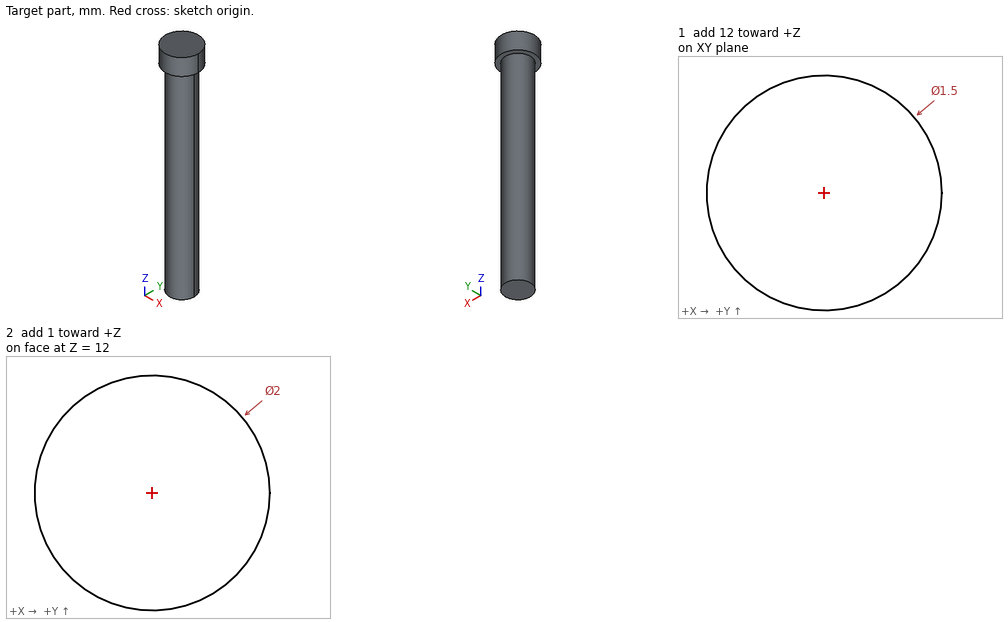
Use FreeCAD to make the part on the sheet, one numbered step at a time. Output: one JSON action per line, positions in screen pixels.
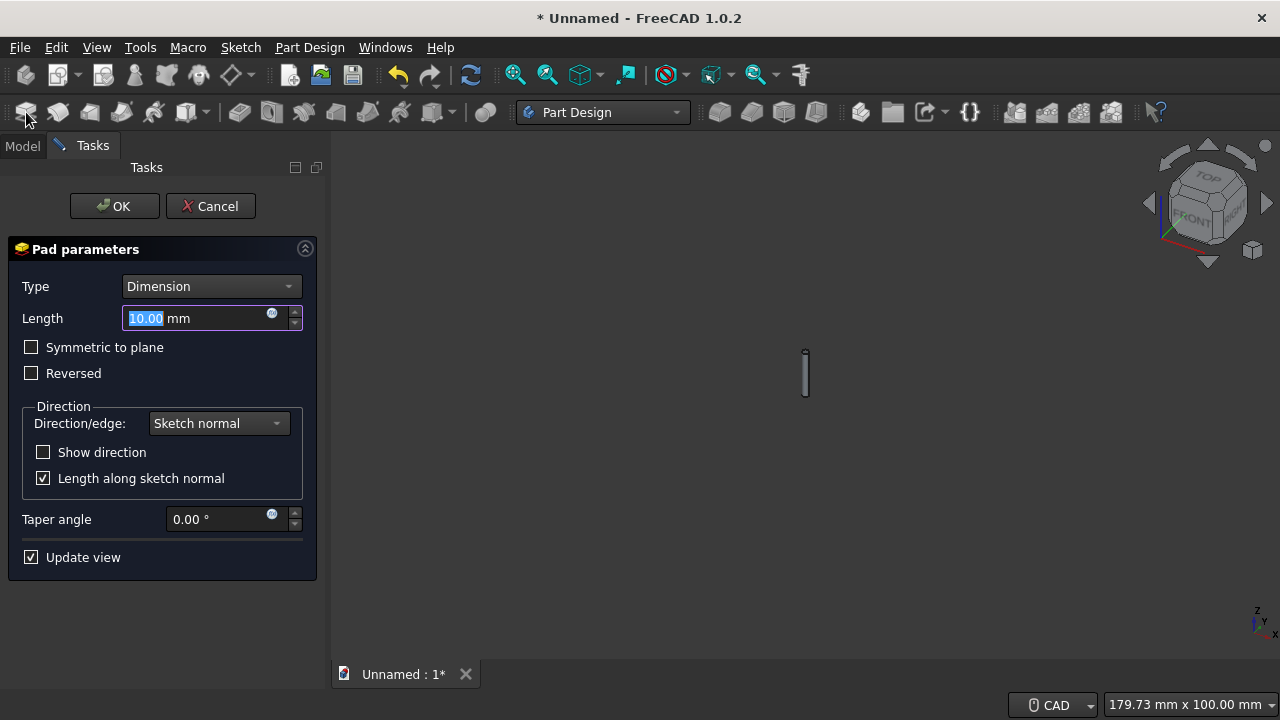
{"action": "type", "text": "12"}
{"action": "key", "text": "Tab"}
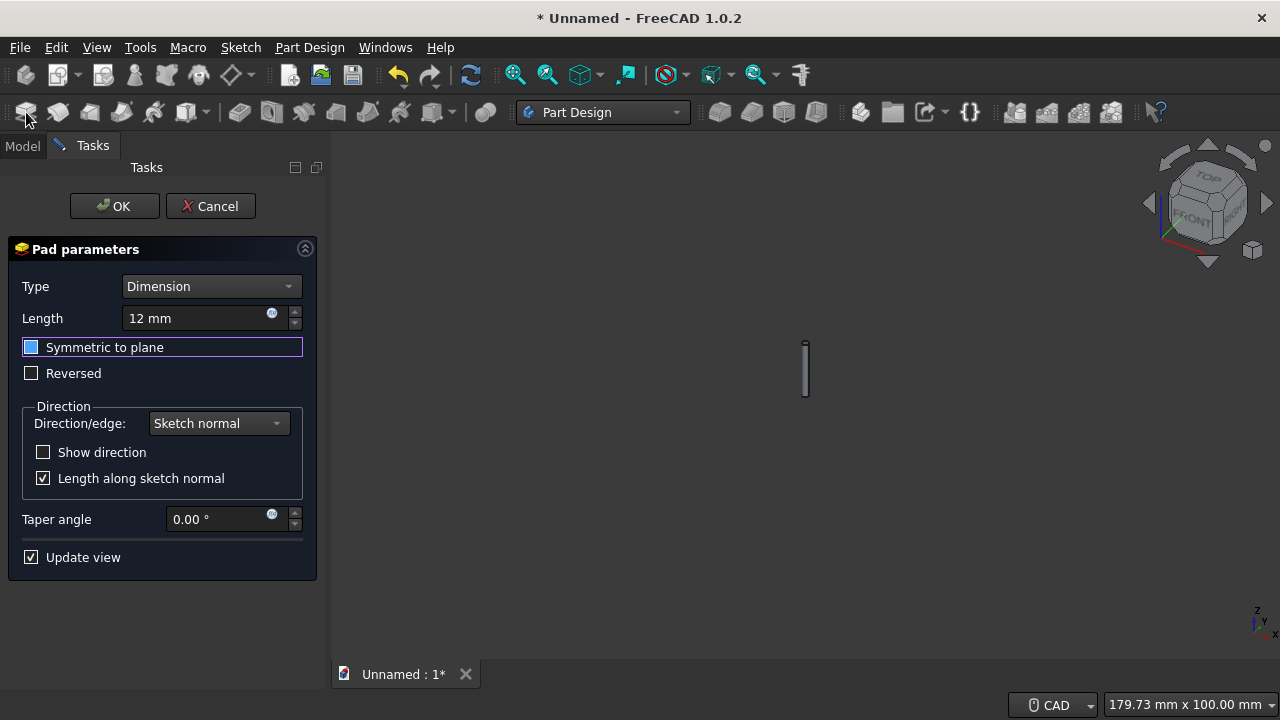
{"action": "left_click", "coordinate": [115, 206]}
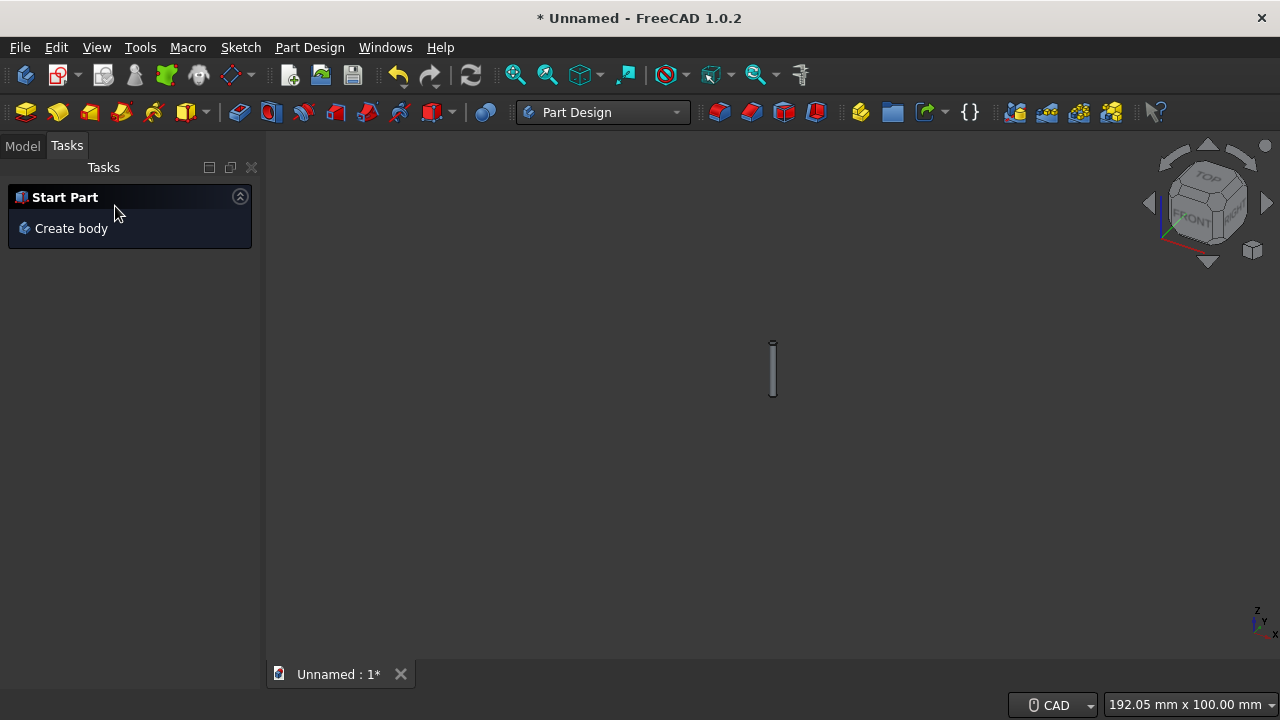
{"action": "left_click", "coordinate": [516, 76]}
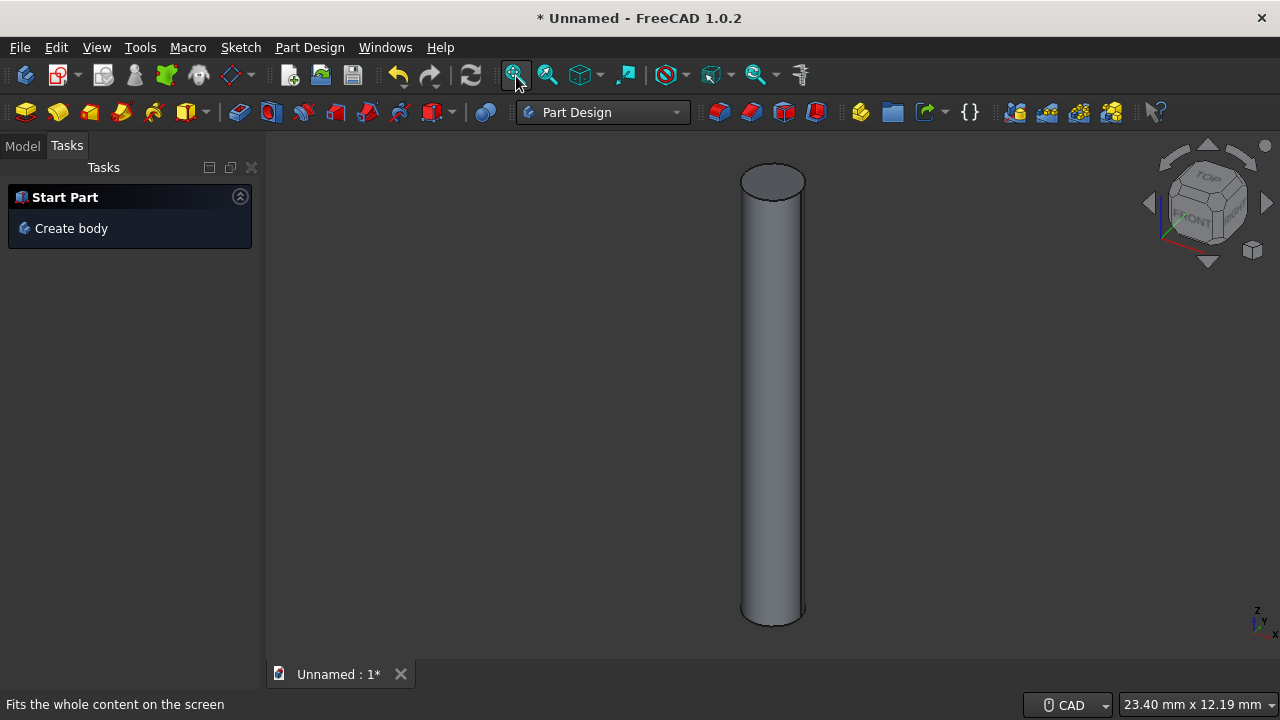
{"action": "left_click", "coordinate": [773, 181]}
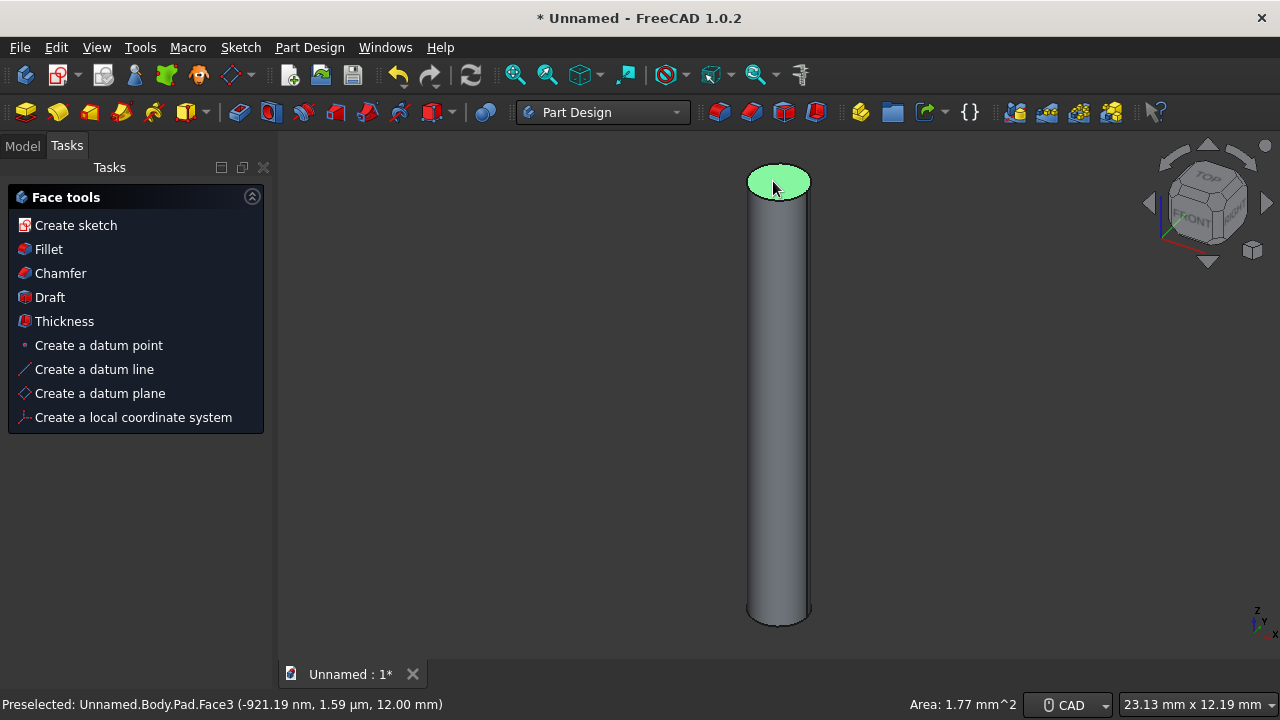
{"action": "left_click", "coordinate": [58, 76]}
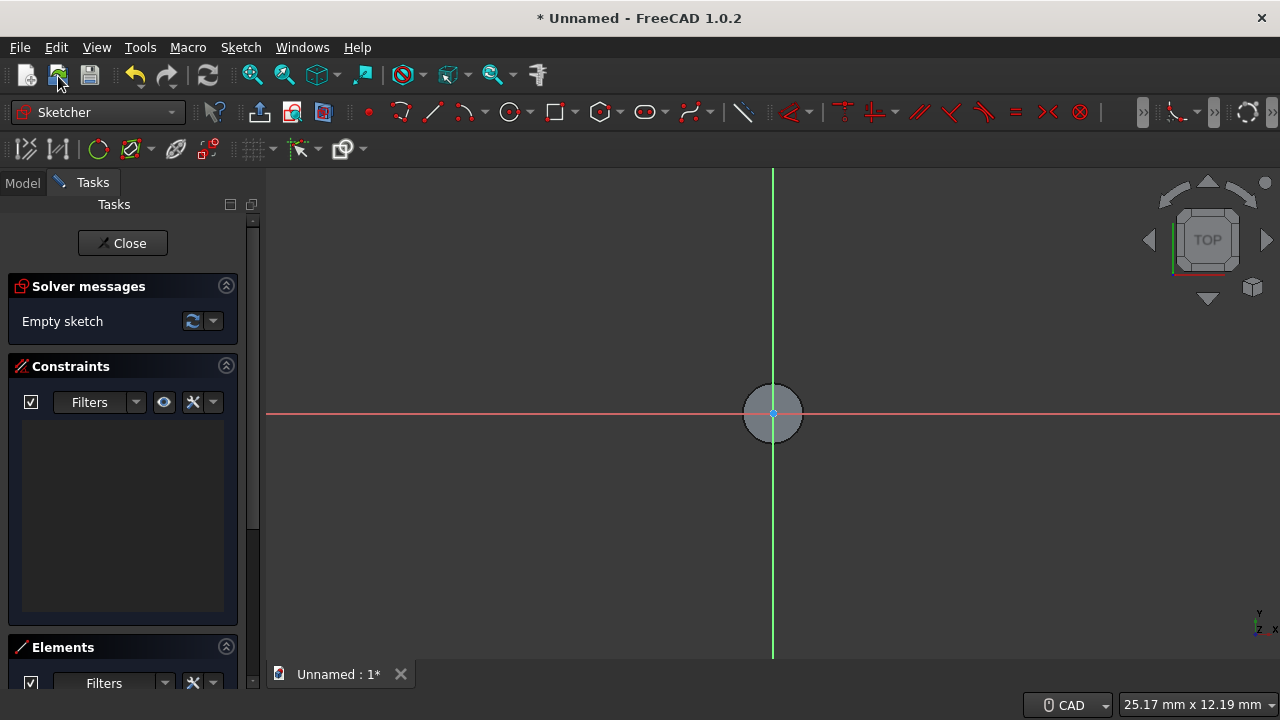
{"action": "scroll", "coordinate": [795, 414], "scroll_direction": "up", "scroll_amount": 7}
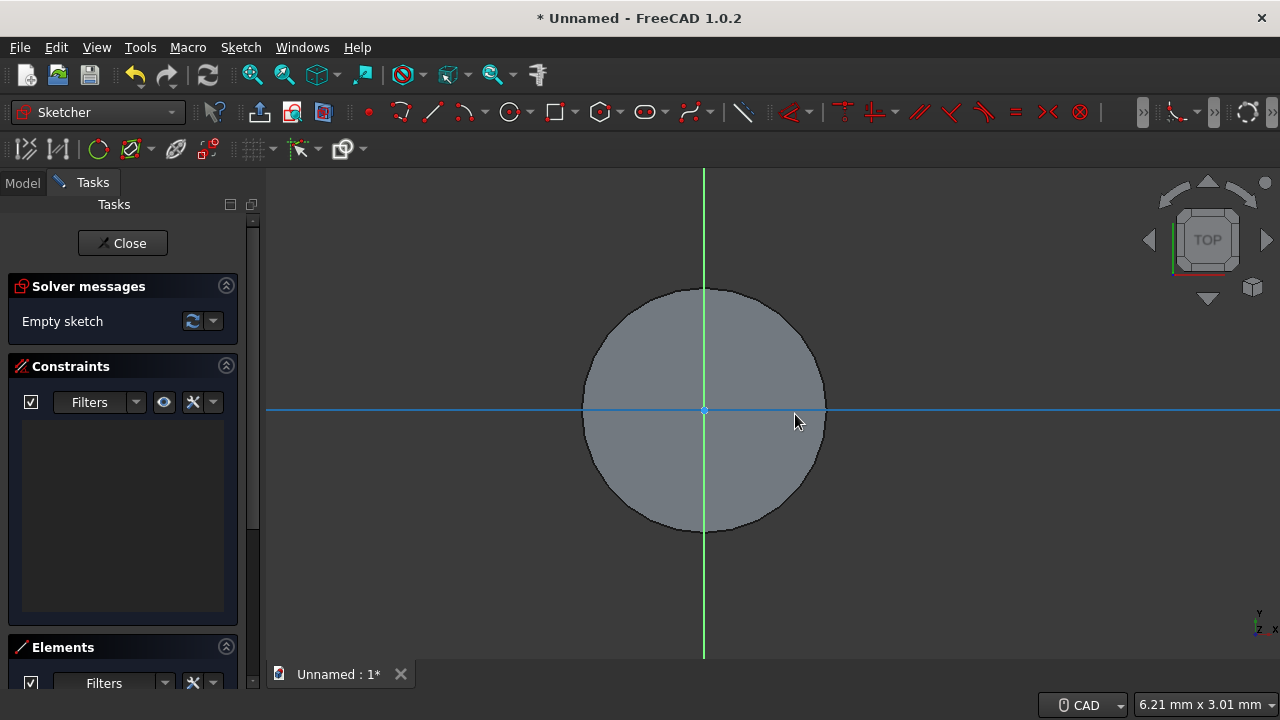
{"action": "left_click", "coordinate": [510, 112]}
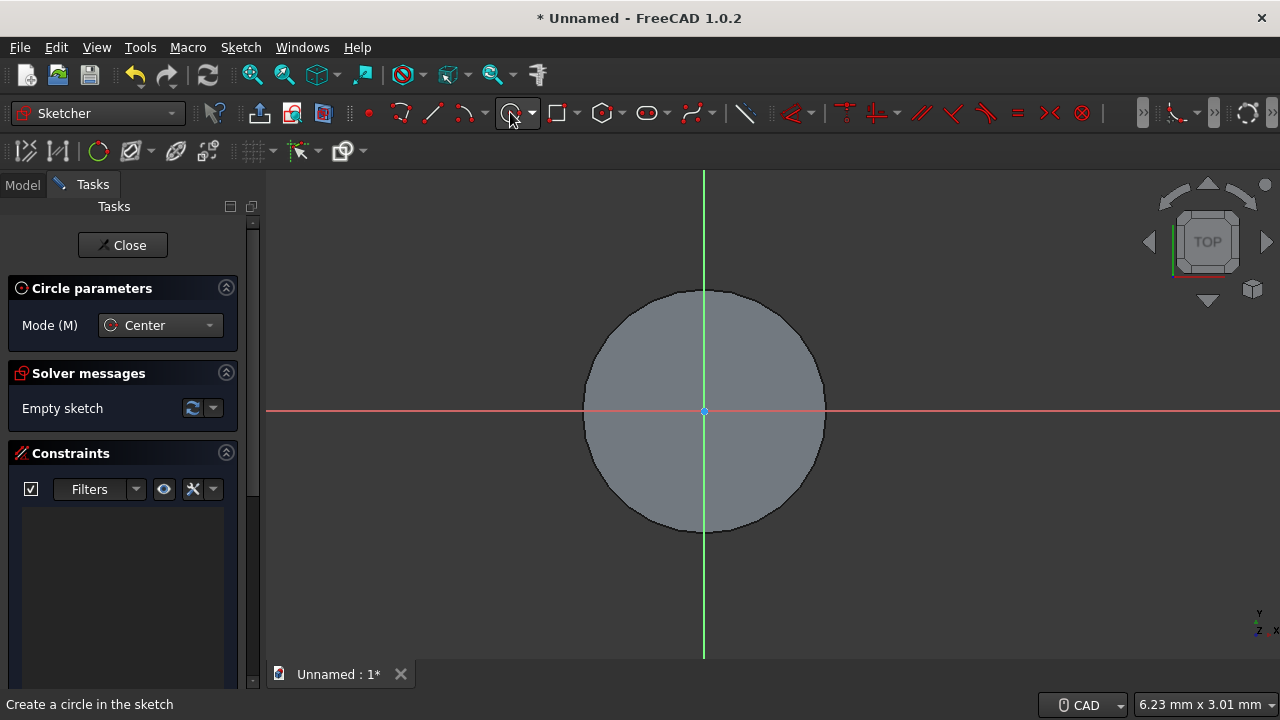
{"action": "left_click", "coordinate": [704, 411]}
{"action": "mouse_move", "coordinate": [820, 296]}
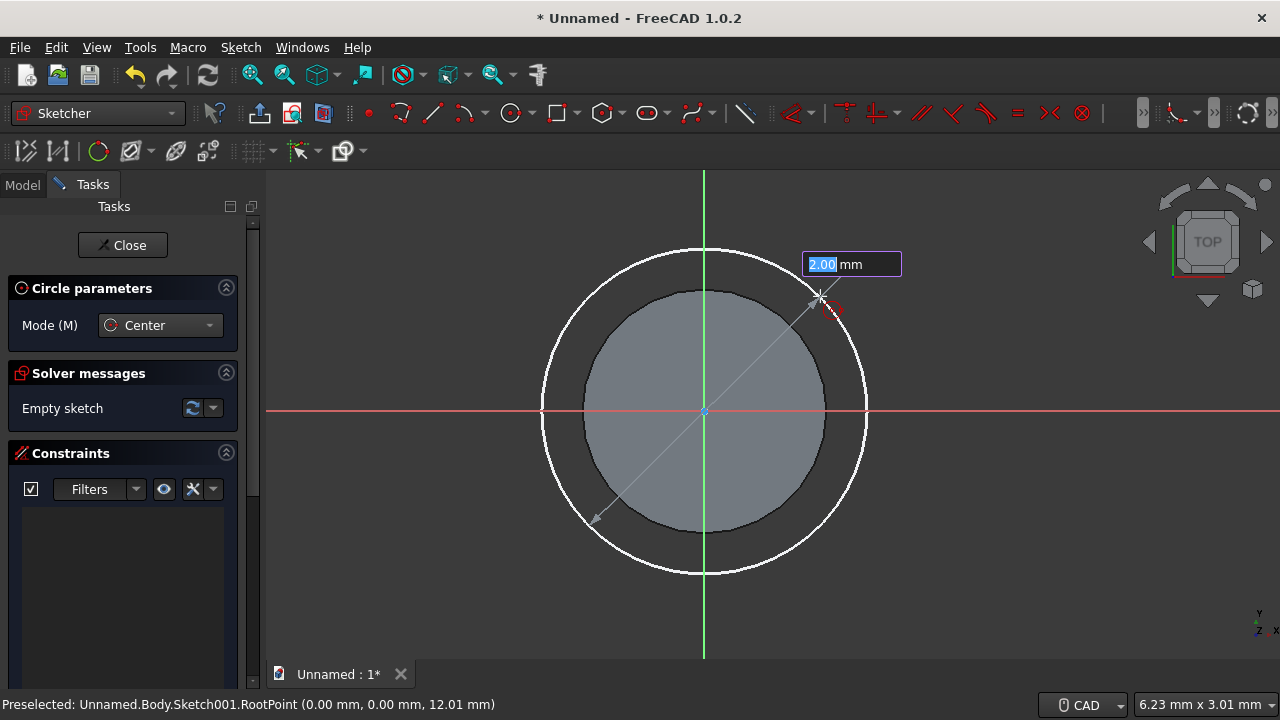
{"action": "type", "text": "2"}
{"action": "key", "text": "Return"}
{"action": "key", "text": "Escape"}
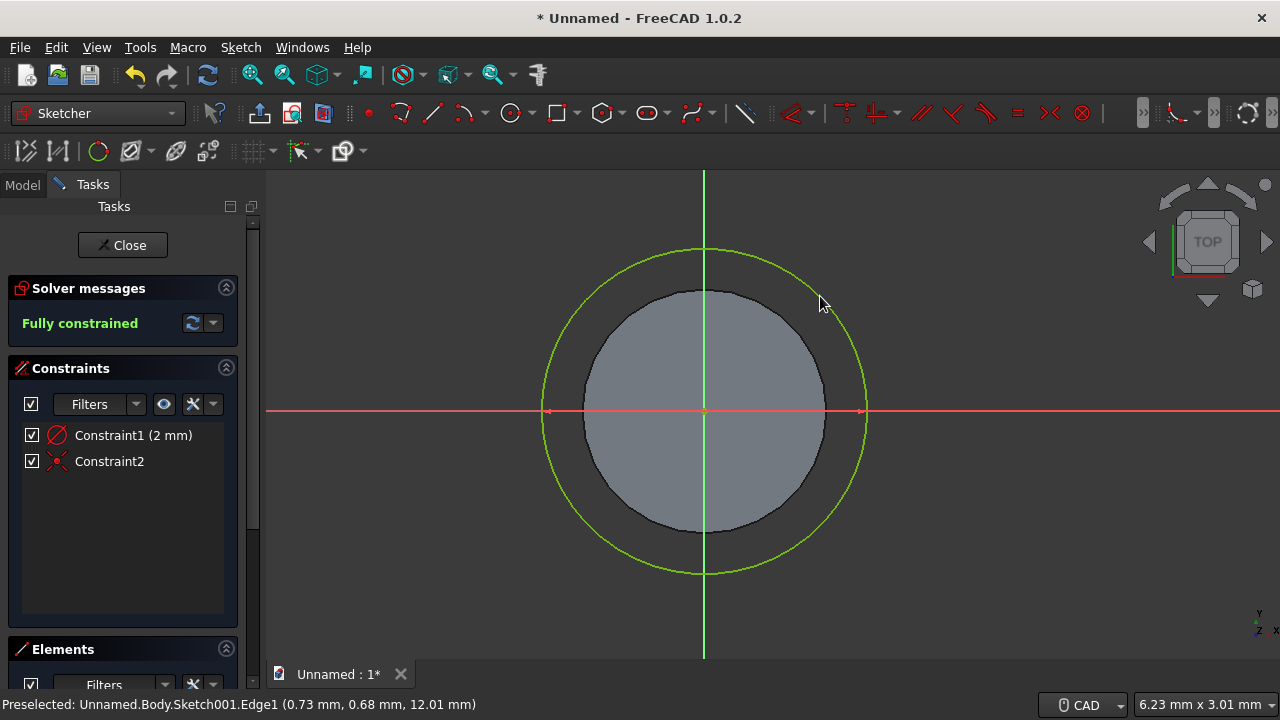
{"action": "left_click", "coordinate": [123, 245]}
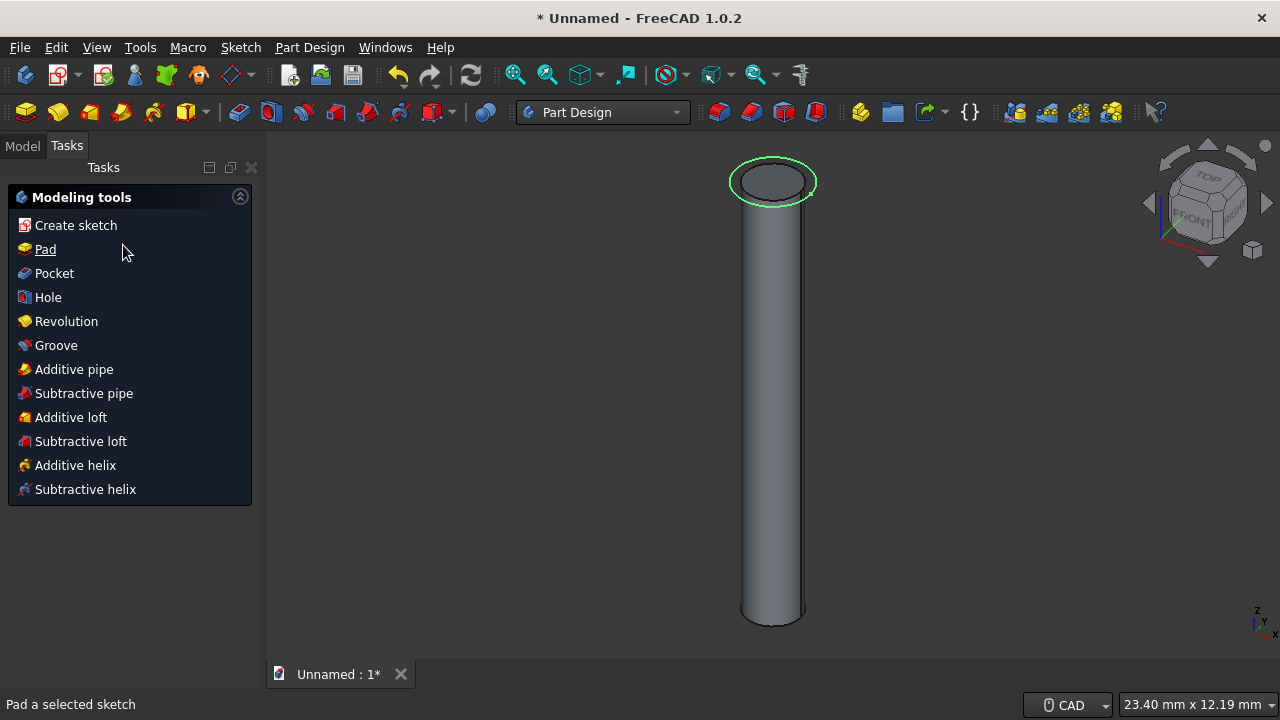
{"action": "left_click", "coordinate": [26, 112]}